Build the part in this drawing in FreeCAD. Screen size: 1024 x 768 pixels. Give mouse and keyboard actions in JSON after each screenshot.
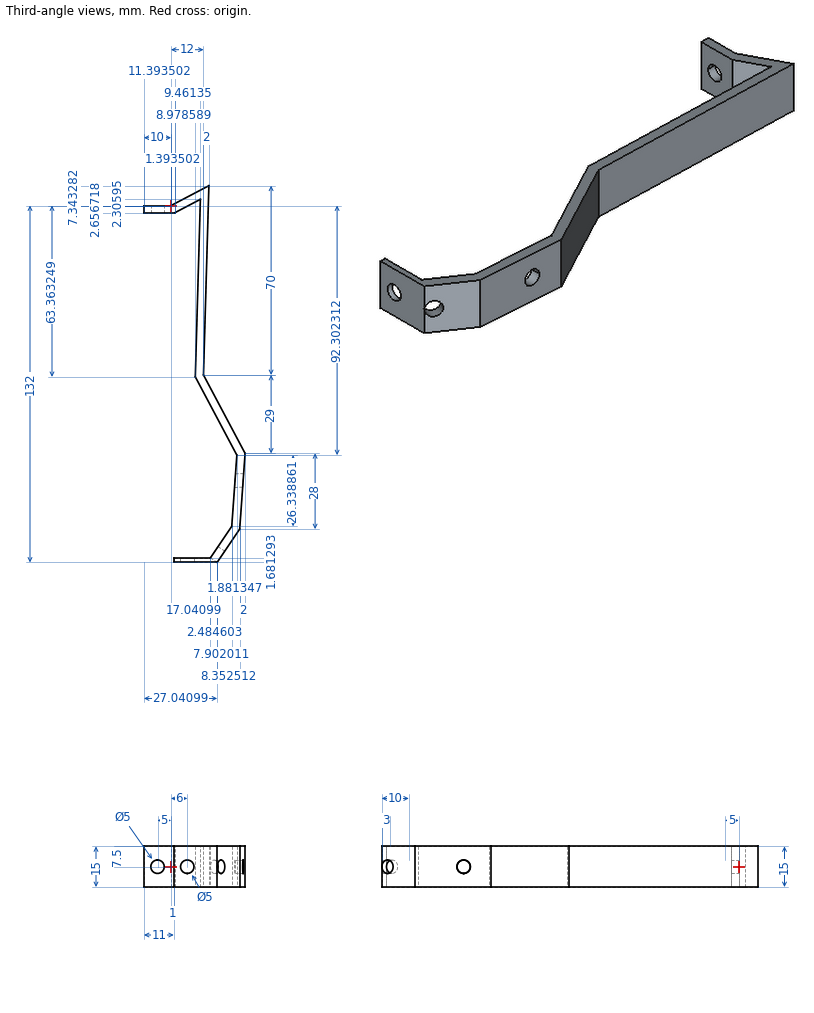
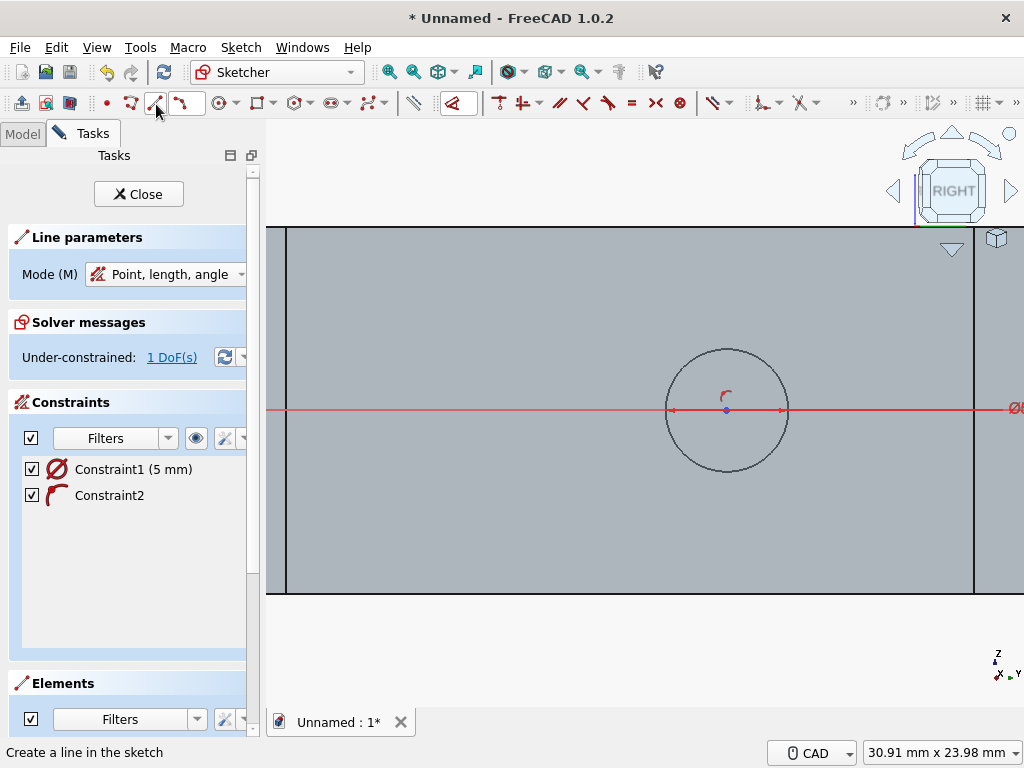
{"action": "left_click", "coordinate": [359, 484]}
{"action": "left_click", "coordinate": [359, 337]}
{"action": "key", "text": "Escape"}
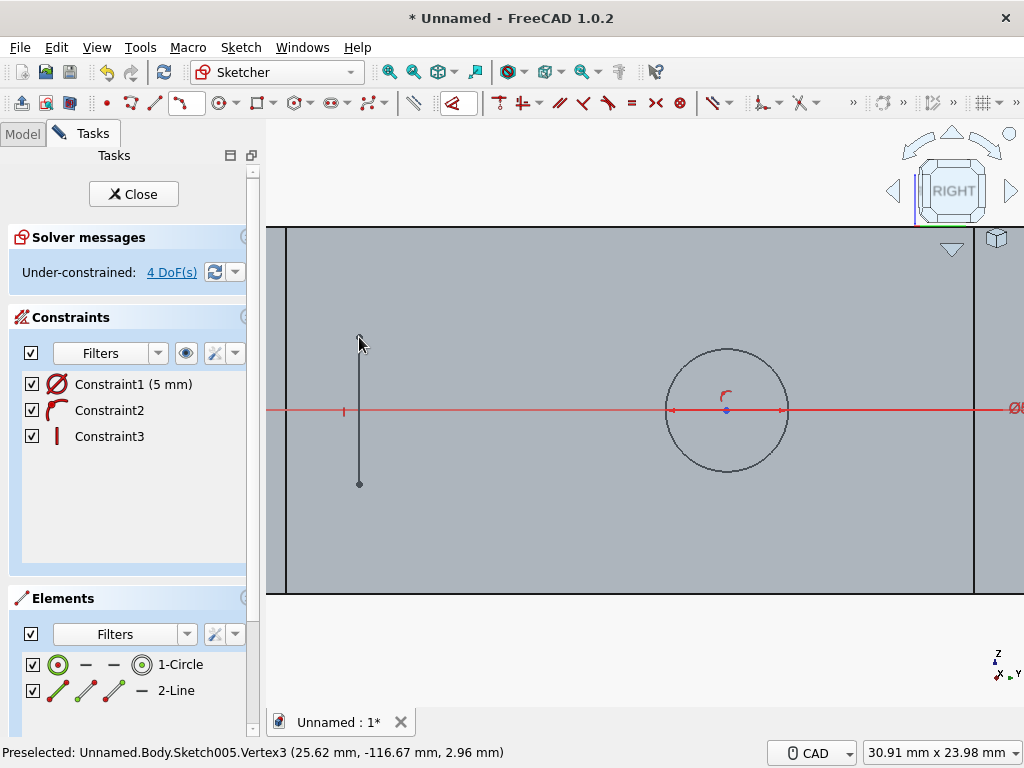
{"action": "left_click", "coordinate": [359, 441]}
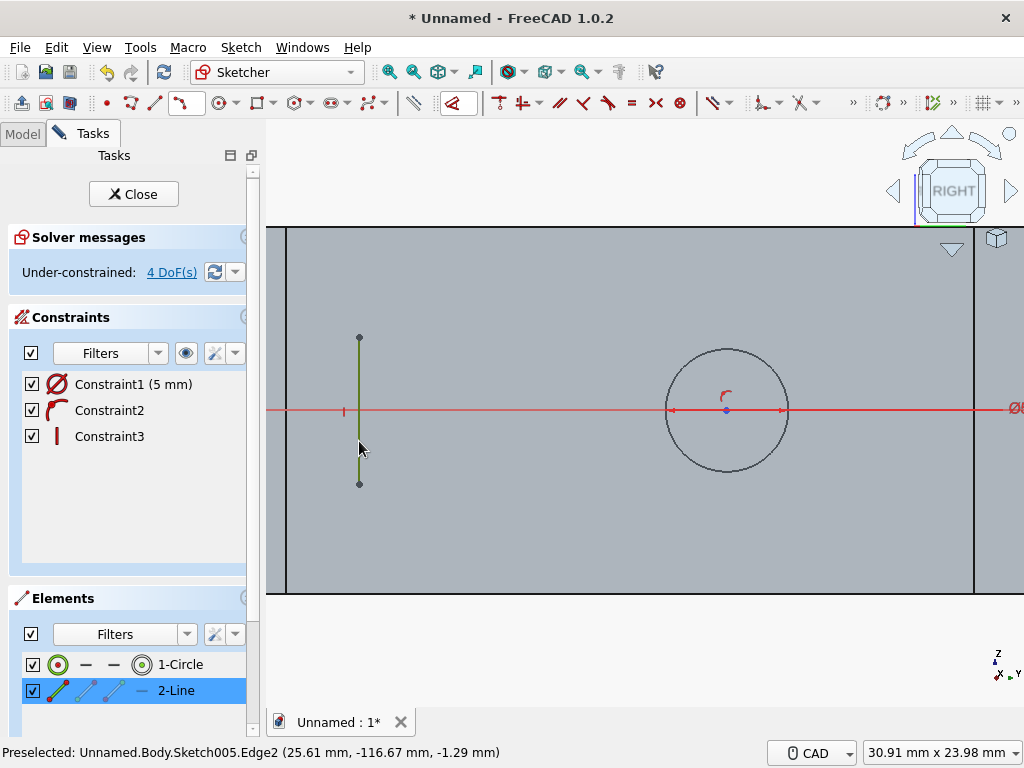
{"action": "left_click", "coordinate": [414, 104]}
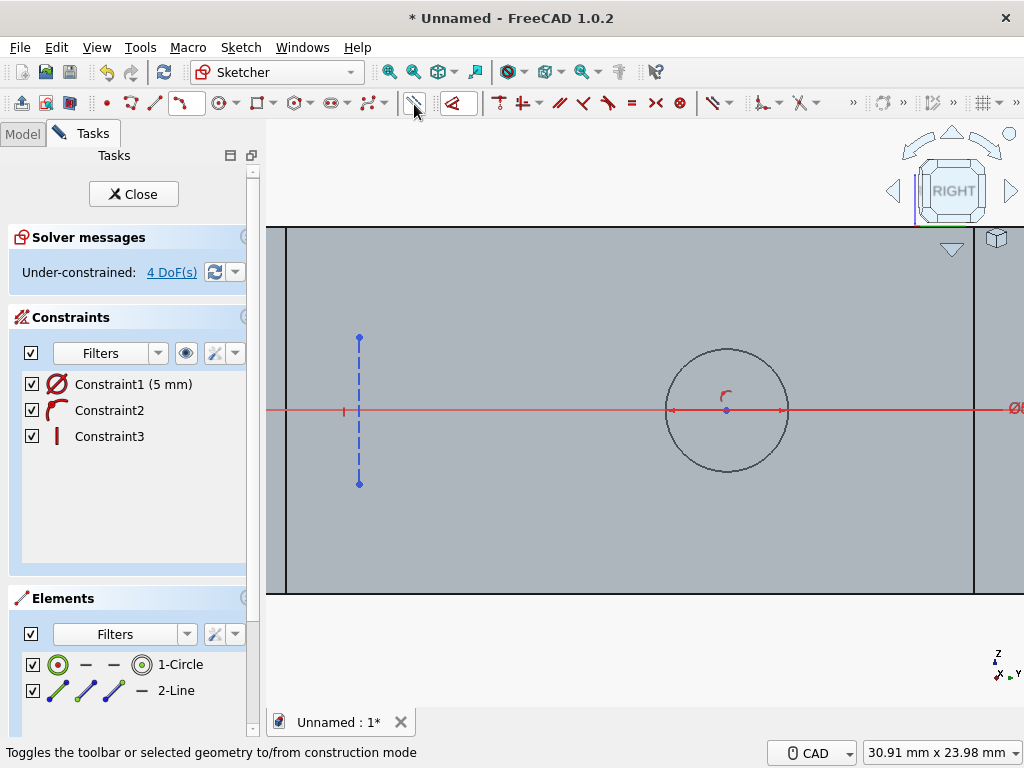
{"action": "left_click", "coordinate": [359, 485]}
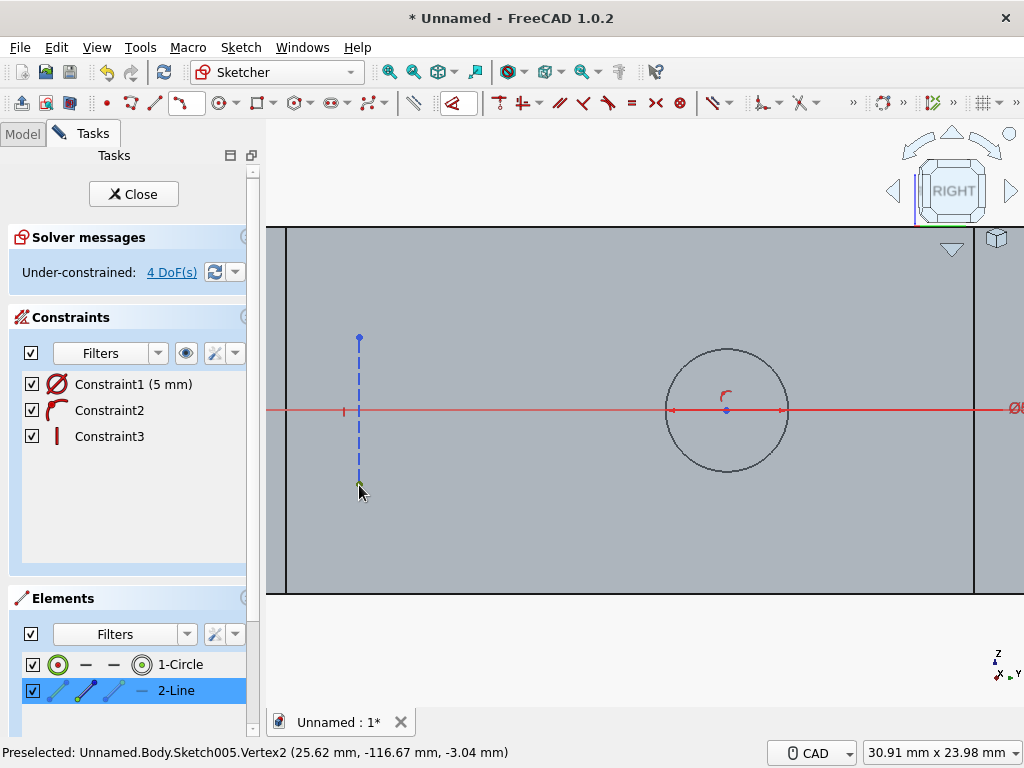
{"action": "left_click", "coordinate": [727, 410]}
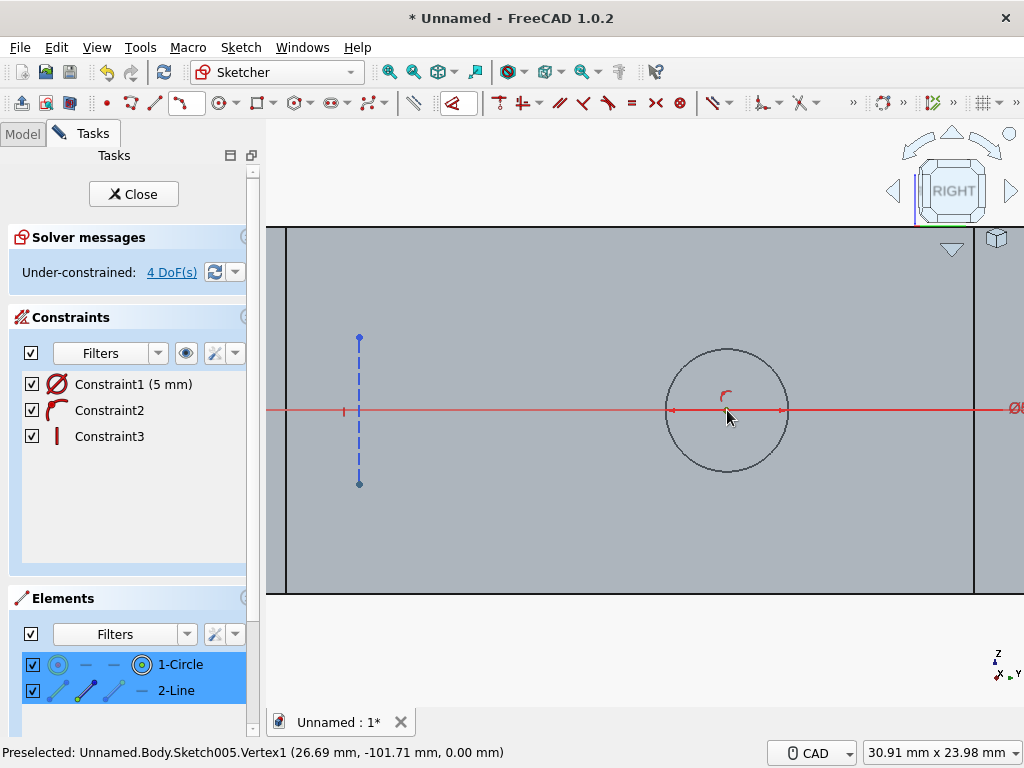
{"action": "key", "text": "l"}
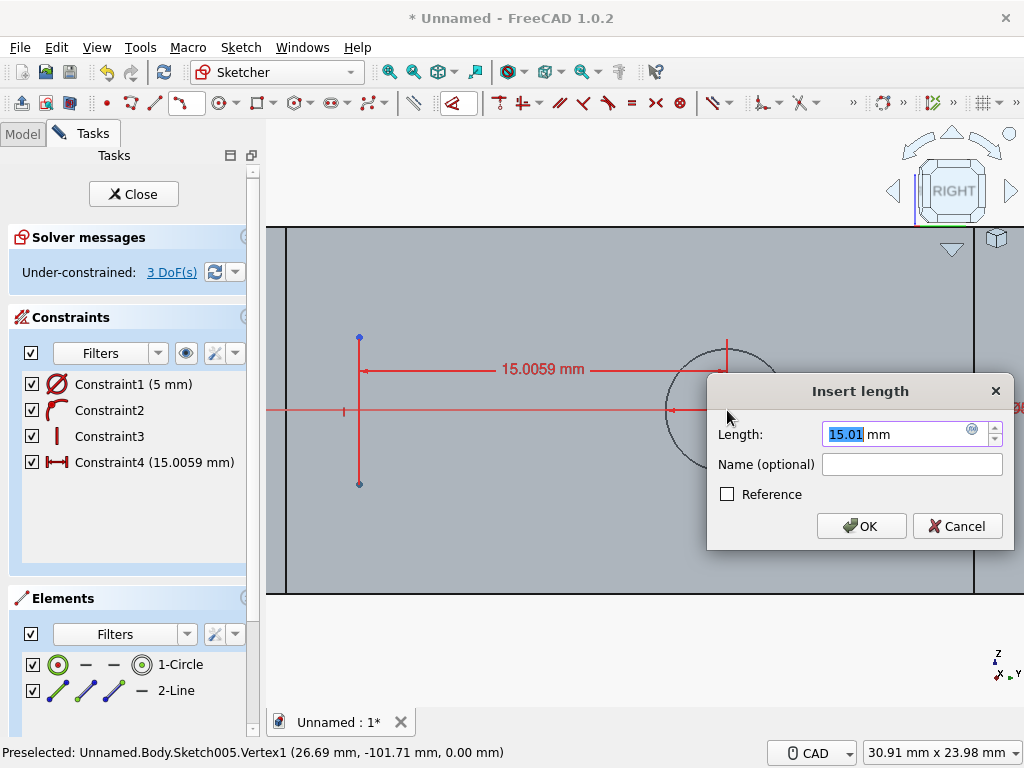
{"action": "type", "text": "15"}
{"action": "key", "text": "Return"}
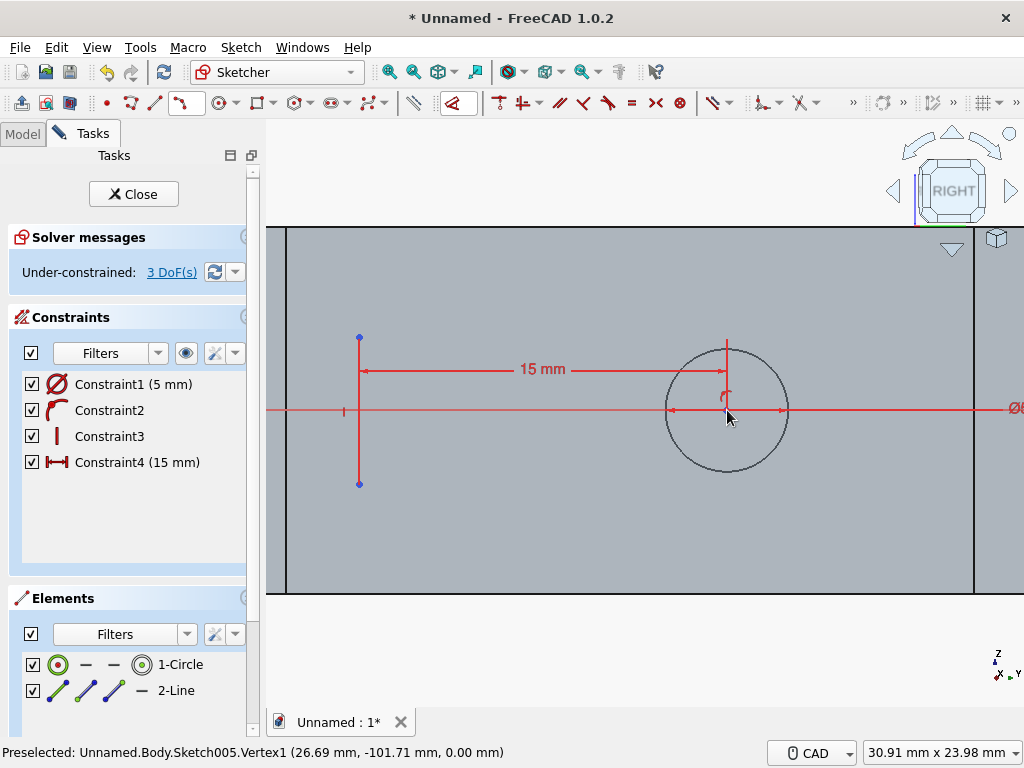
{"action": "left_click", "coordinate": [727, 410]}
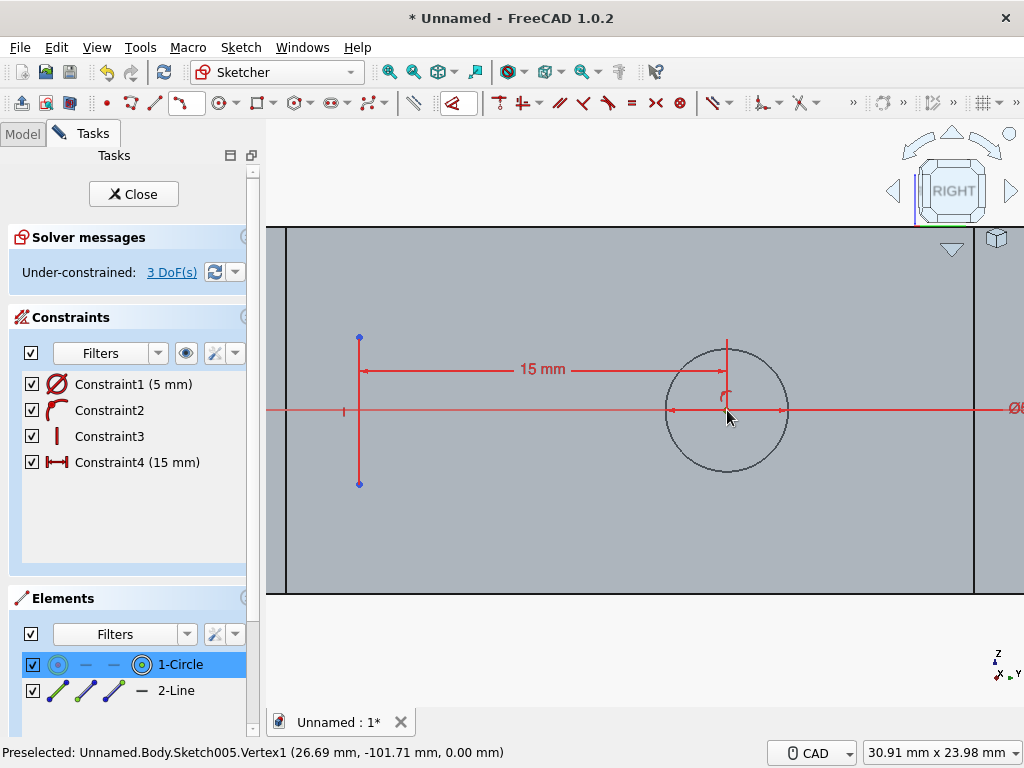
{"action": "left_click", "coordinate": [472, 104]}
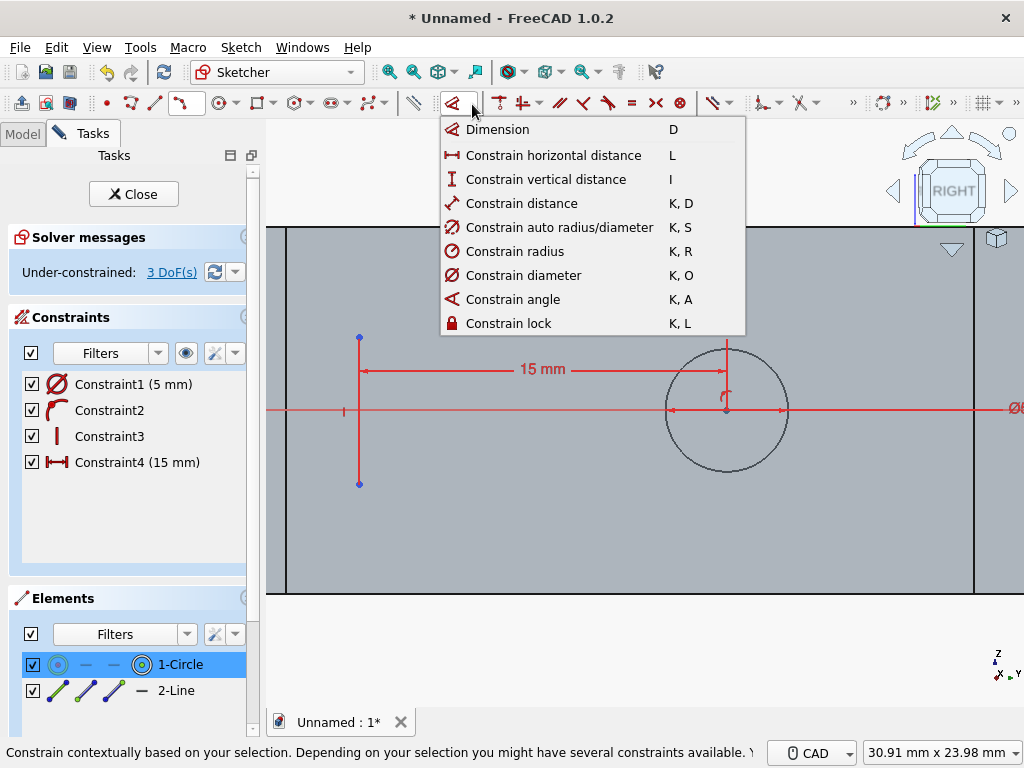
{"action": "left_click", "coordinate": [593, 155]}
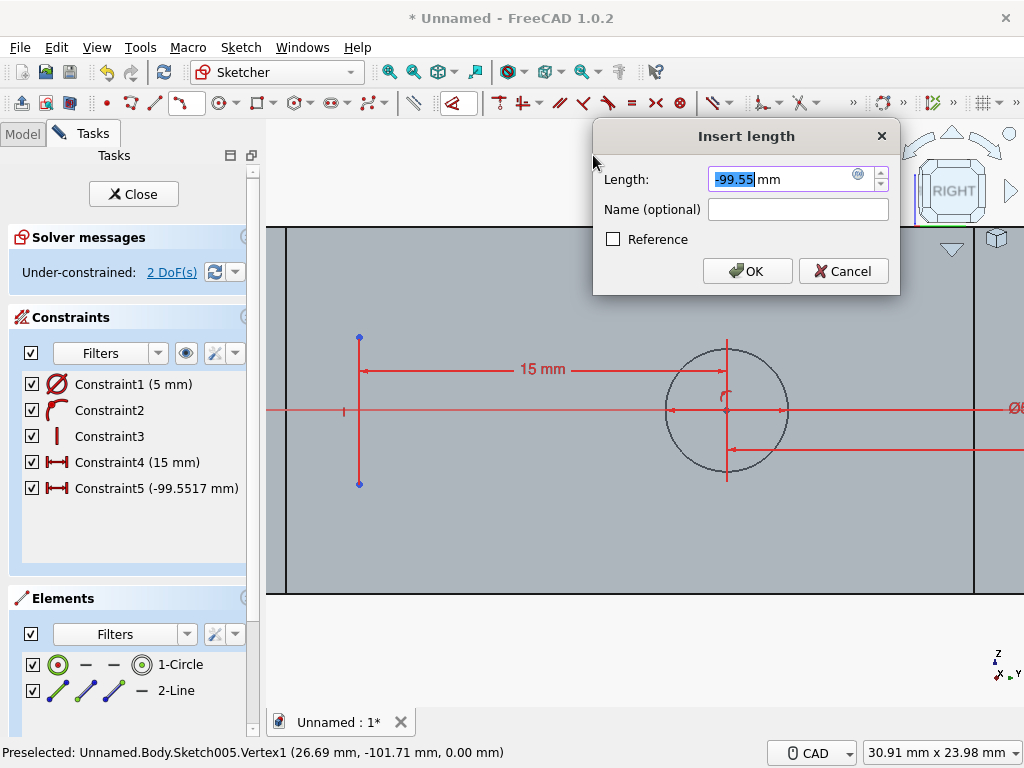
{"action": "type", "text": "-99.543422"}
{"action": "key", "text": "Return"}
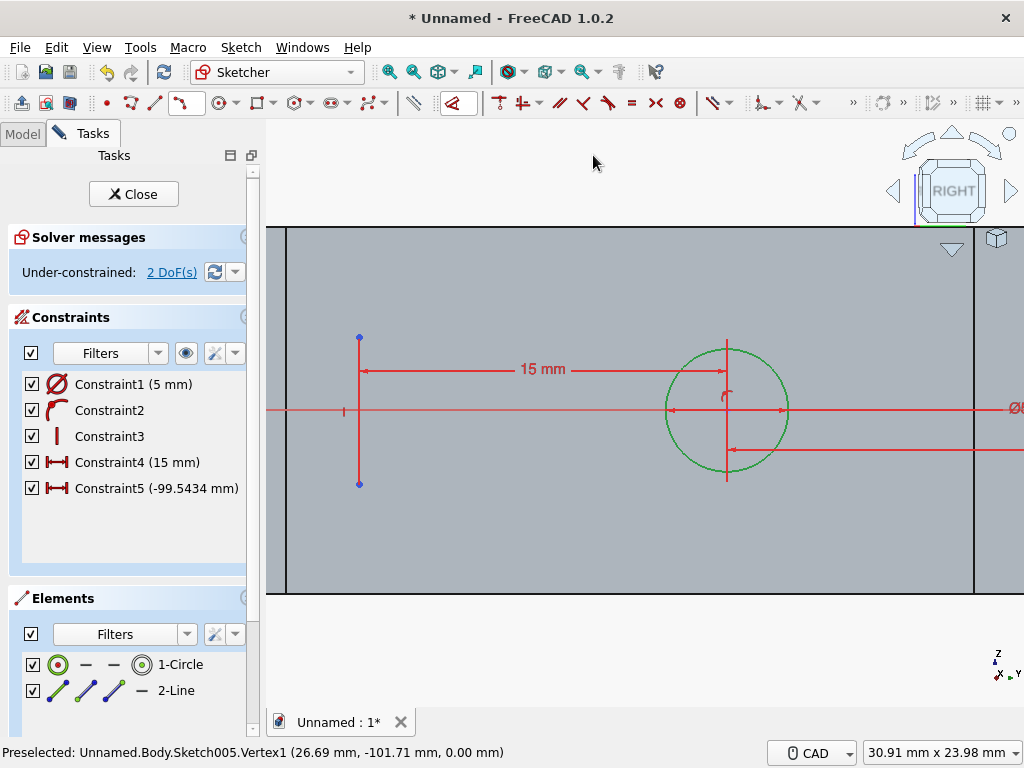
{"action": "left_click", "coordinate": [134, 194]}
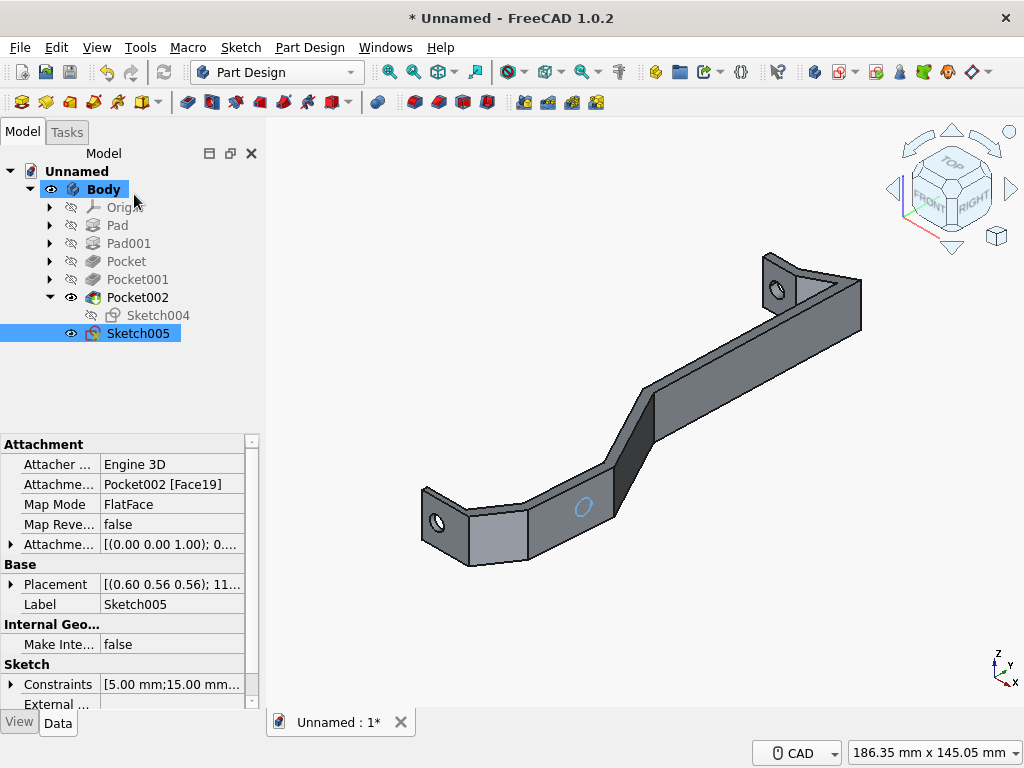
{"action": "left_click", "coordinate": [236, 102]}